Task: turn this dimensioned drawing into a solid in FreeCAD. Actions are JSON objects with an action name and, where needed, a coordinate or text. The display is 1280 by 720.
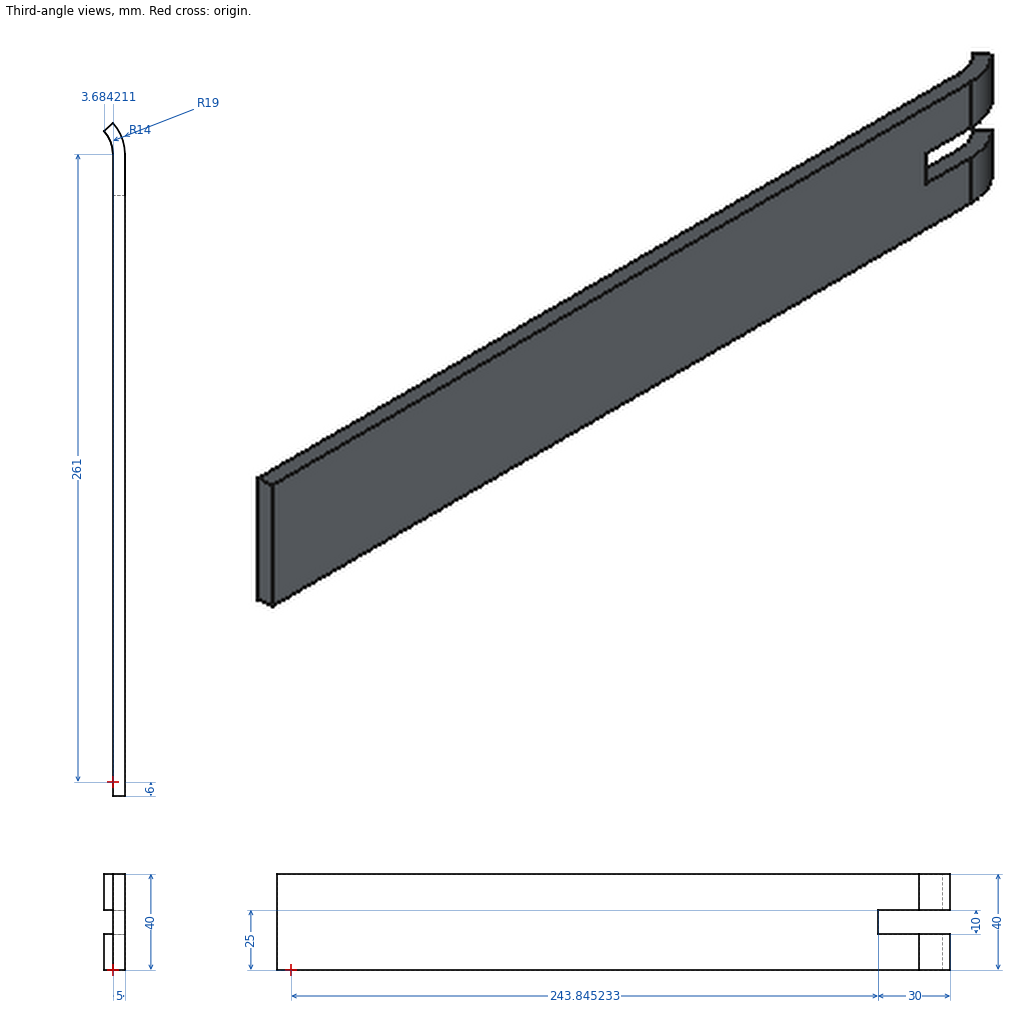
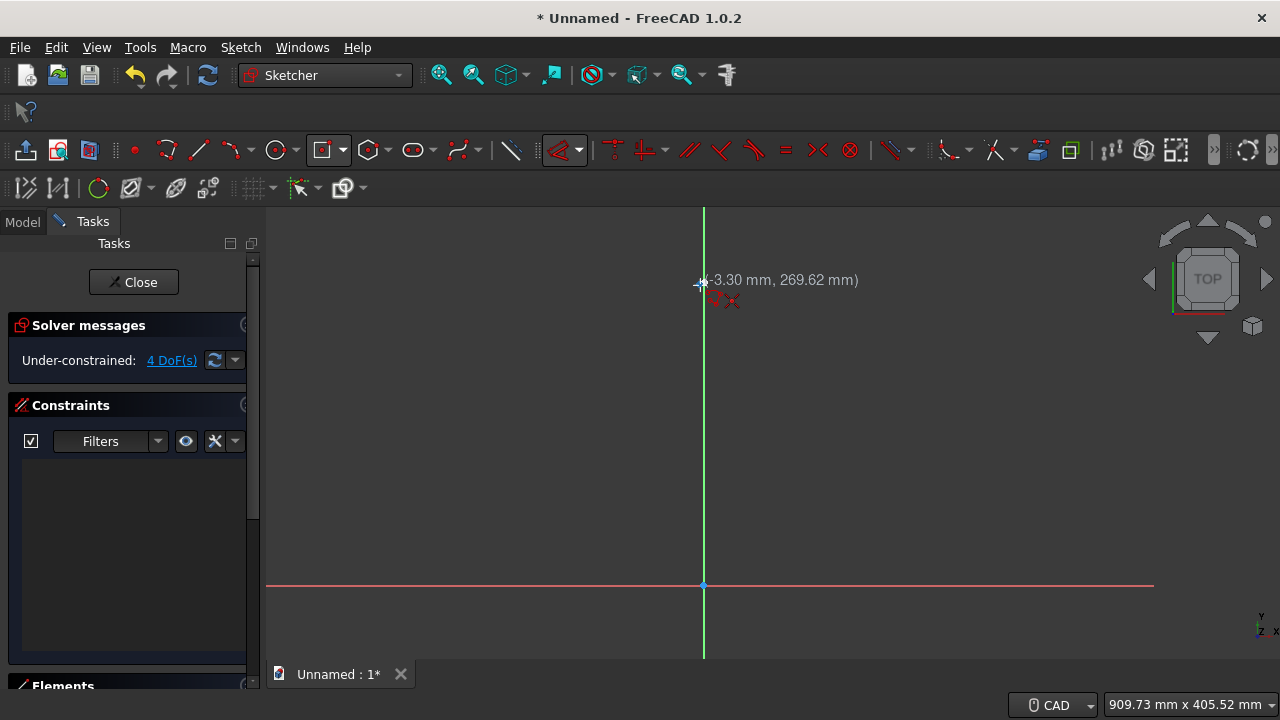
{"action": "scroll", "coordinate": [704, 295], "scroll_direction": "up", "scroll_amount": 2}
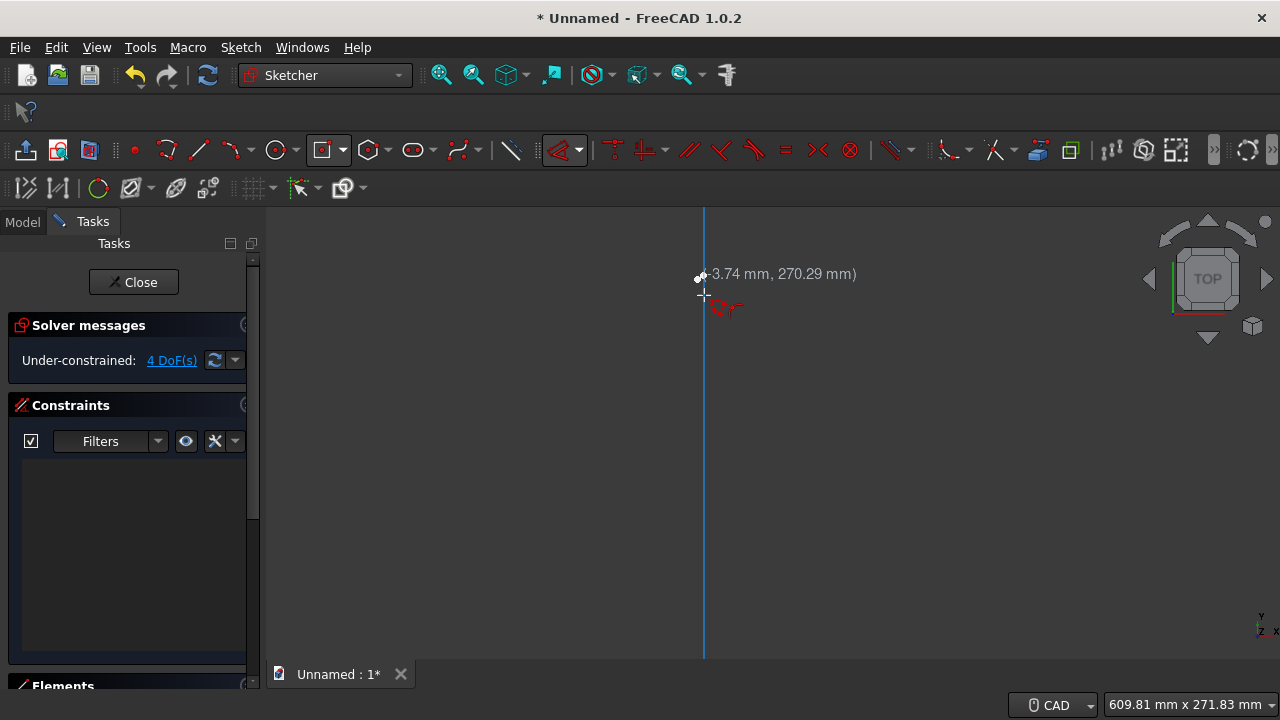
{"action": "left_click", "coordinate": [704, 295]}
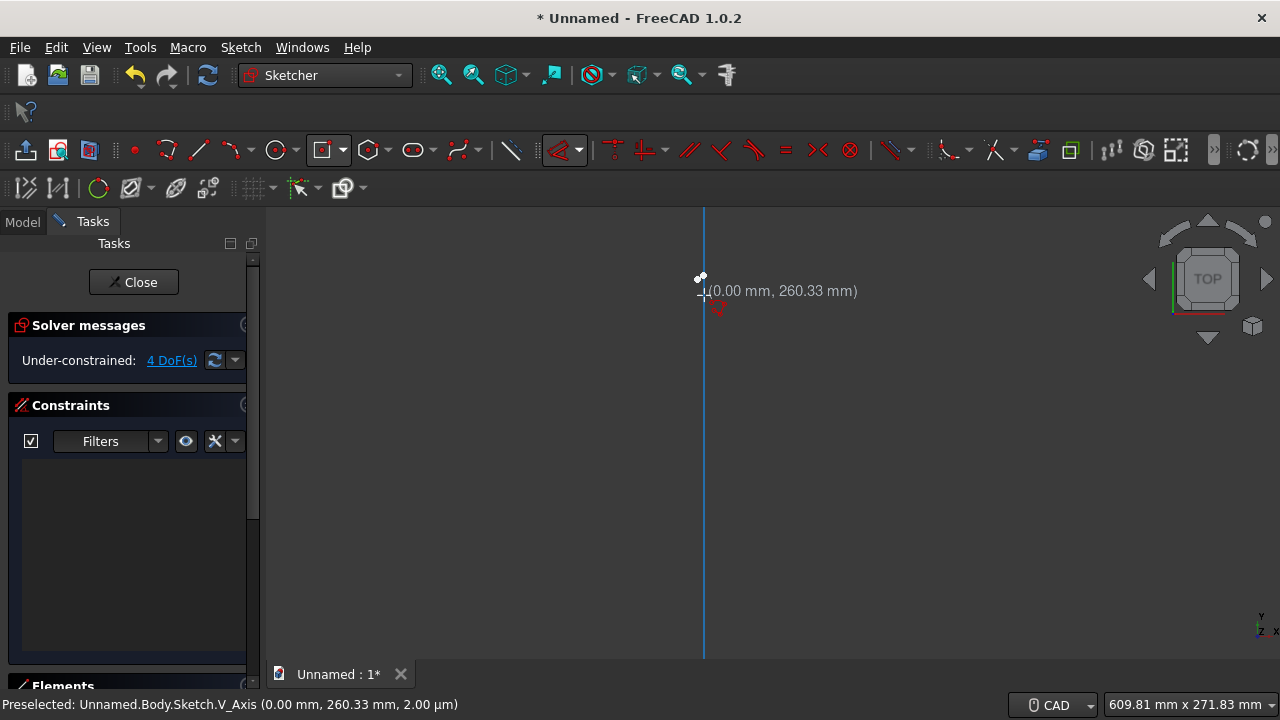
{"action": "scroll", "coordinate": [704, 294], "scroll_direction": "down", "scroll_amount": 2}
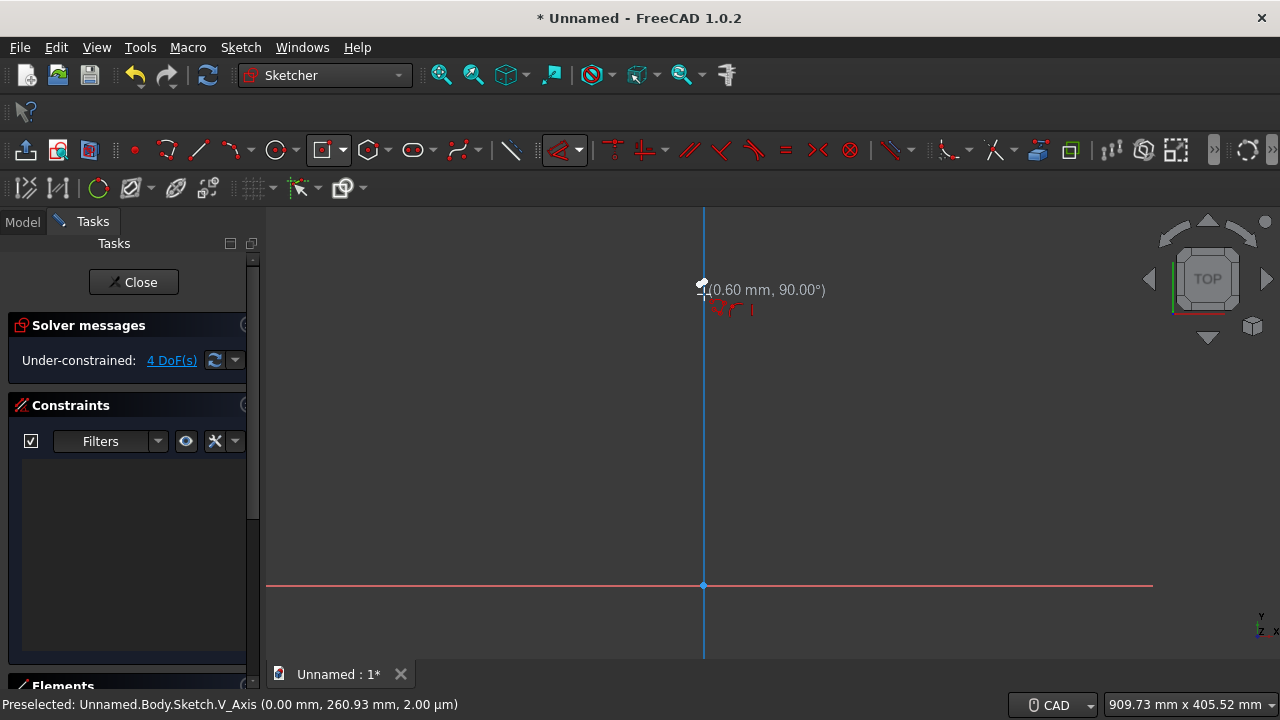
{"action": "left_click", "coordinate": [704, 586]}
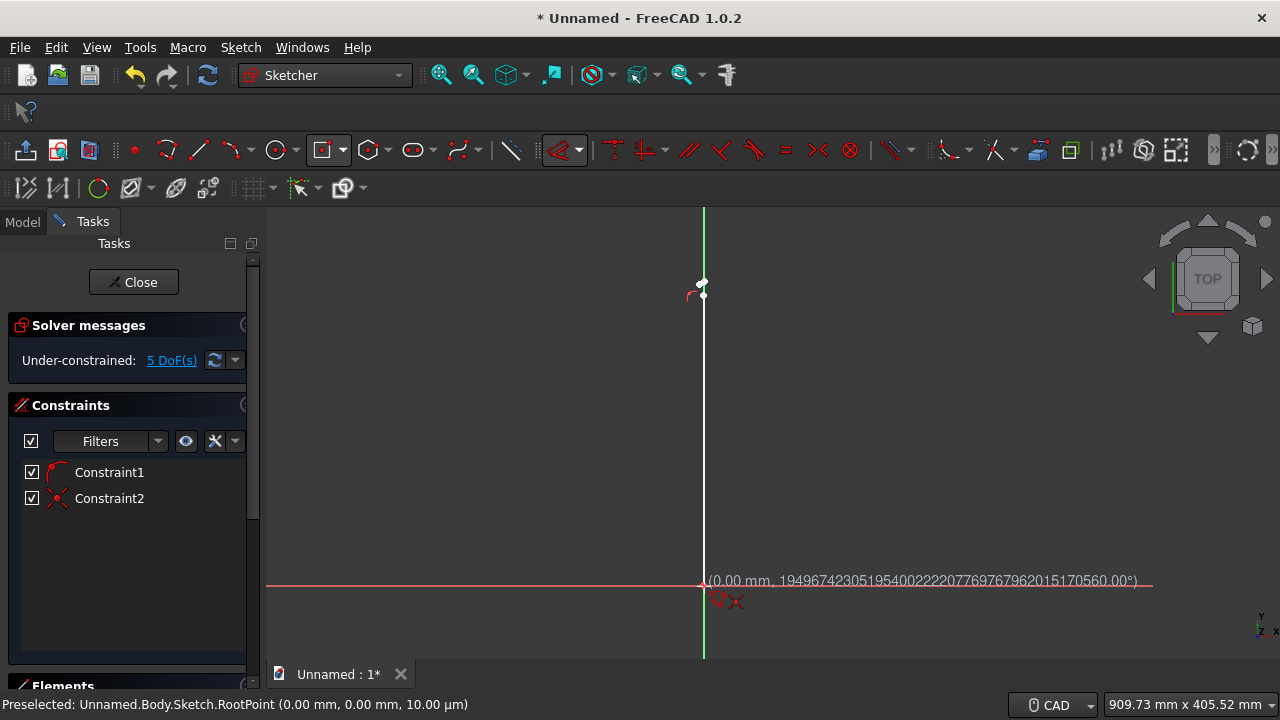
{"action": "scroll", "coordinate": [710, 586], "scroll_direction": "up", "scroll_amount": 6}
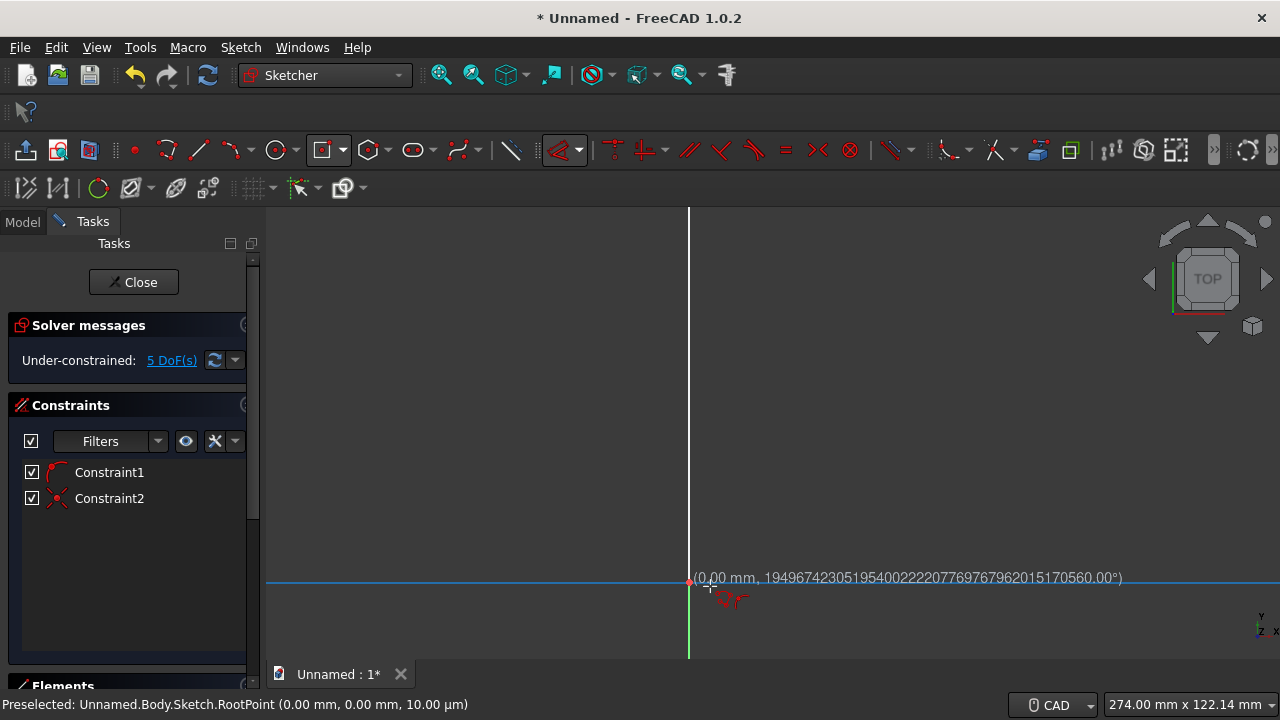
{"action": "left_click", "coordinate": [708, 574]}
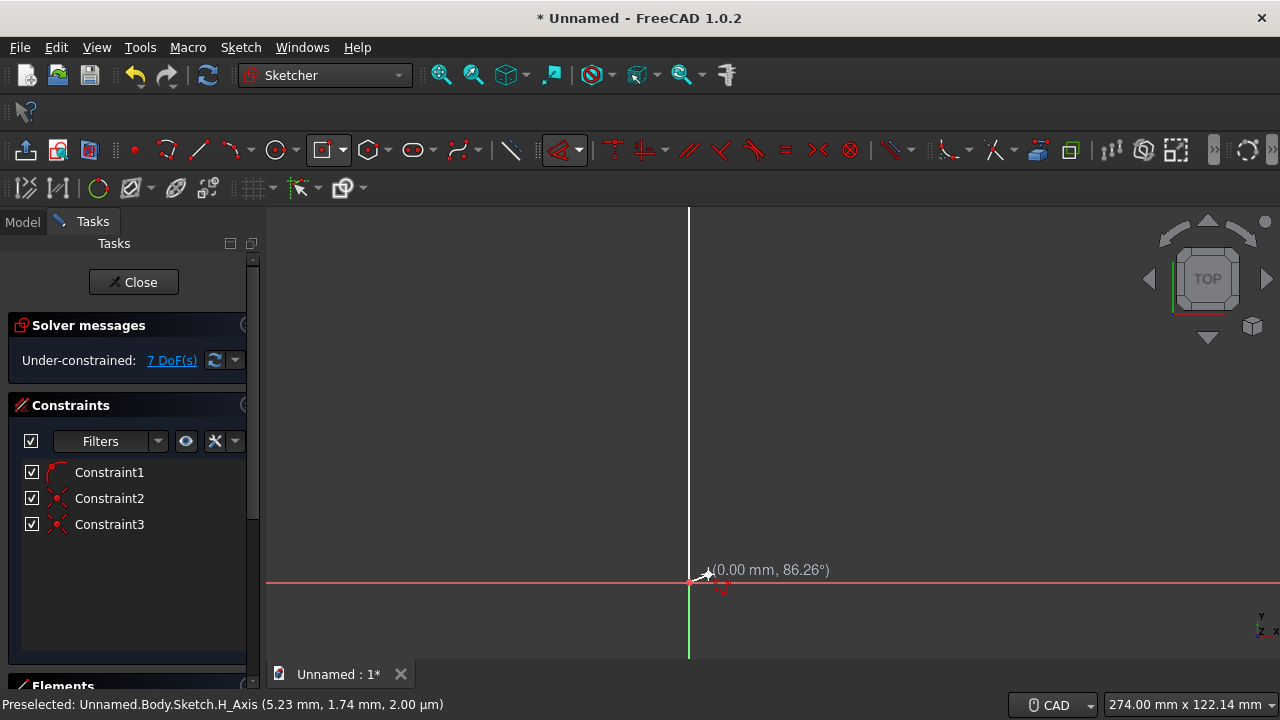
{"action": "scroll", "coordinate": [710, 587], "scroll_direction": "down", "scroll_amount": 6}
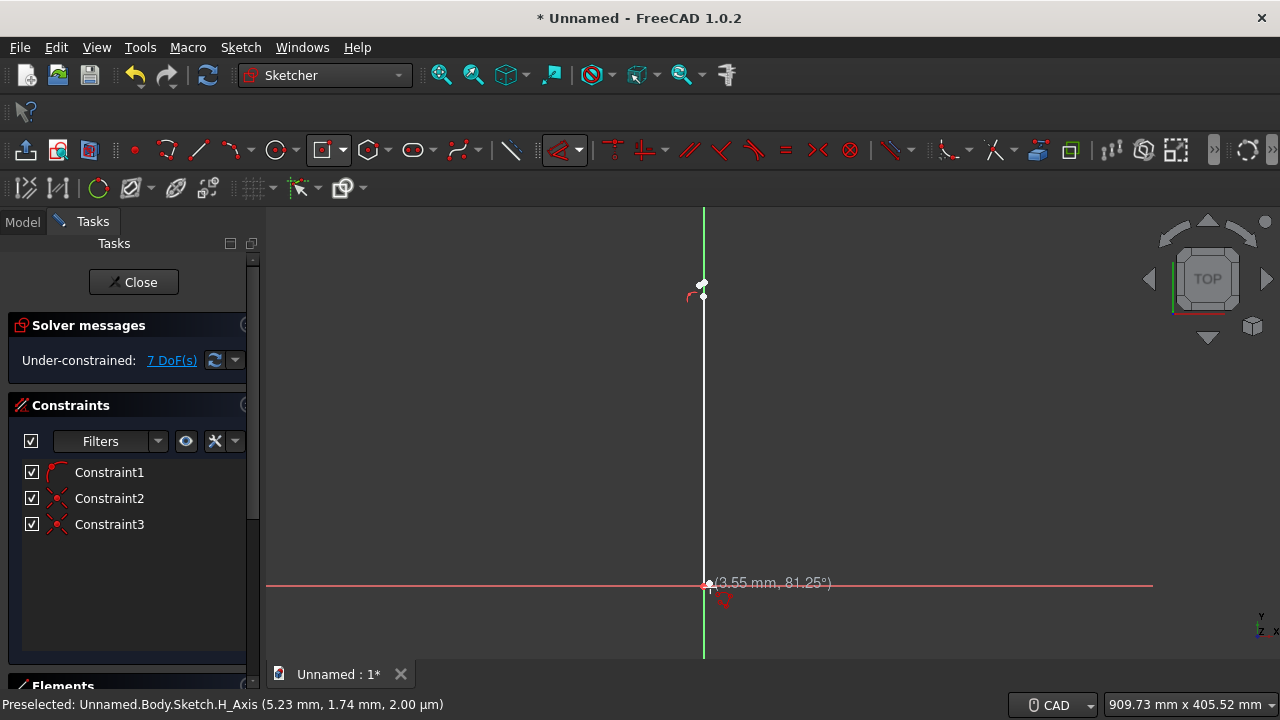
{"action": "scroll", "coordinate": [710, 295], "scroll_direction": "up", "scroll_amount": 6}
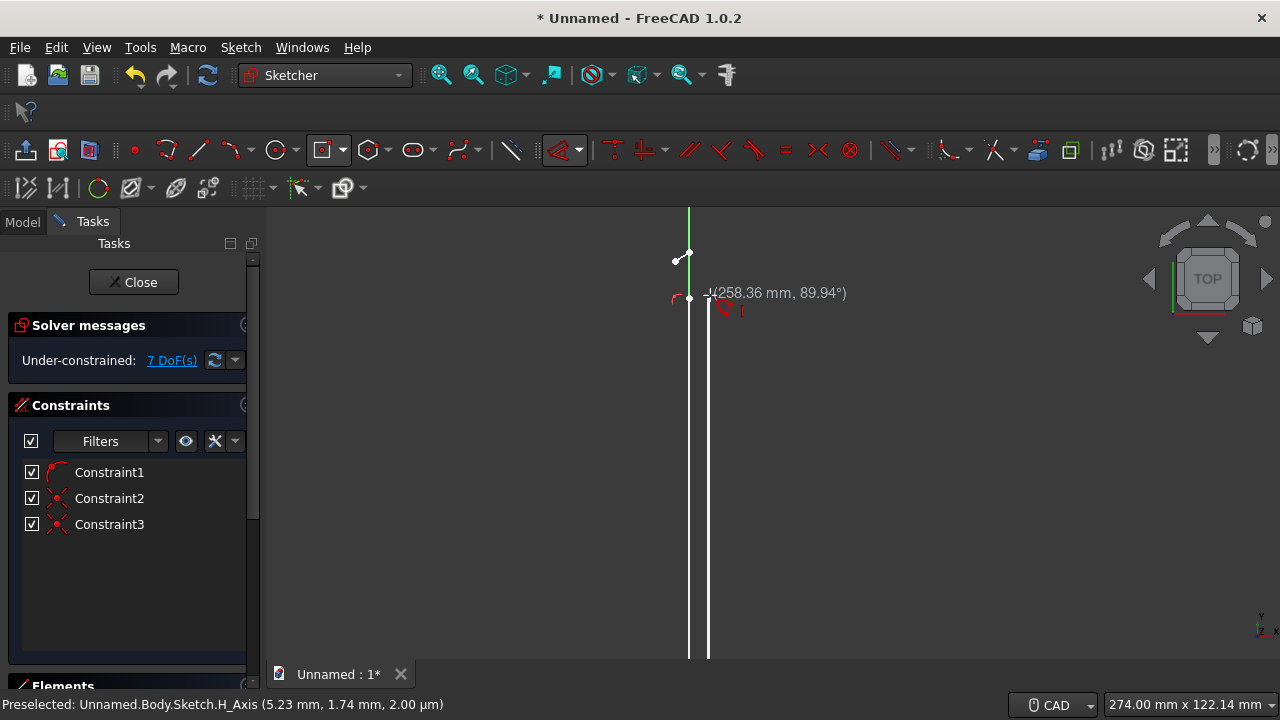
{"action": "left_click", "coordinate": [708, 296]}
{"action": "right_click", "coordinate": [708, 296]}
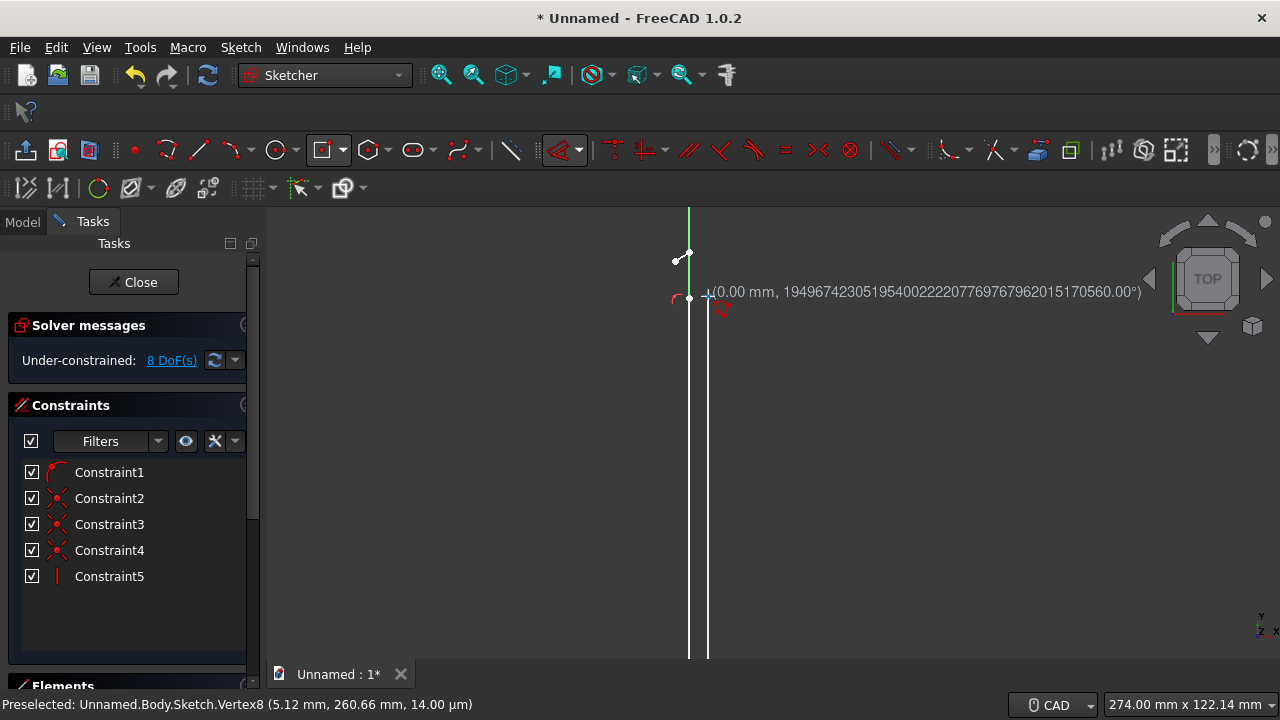
{"action": "left_click", "coordinate": [232, 150]}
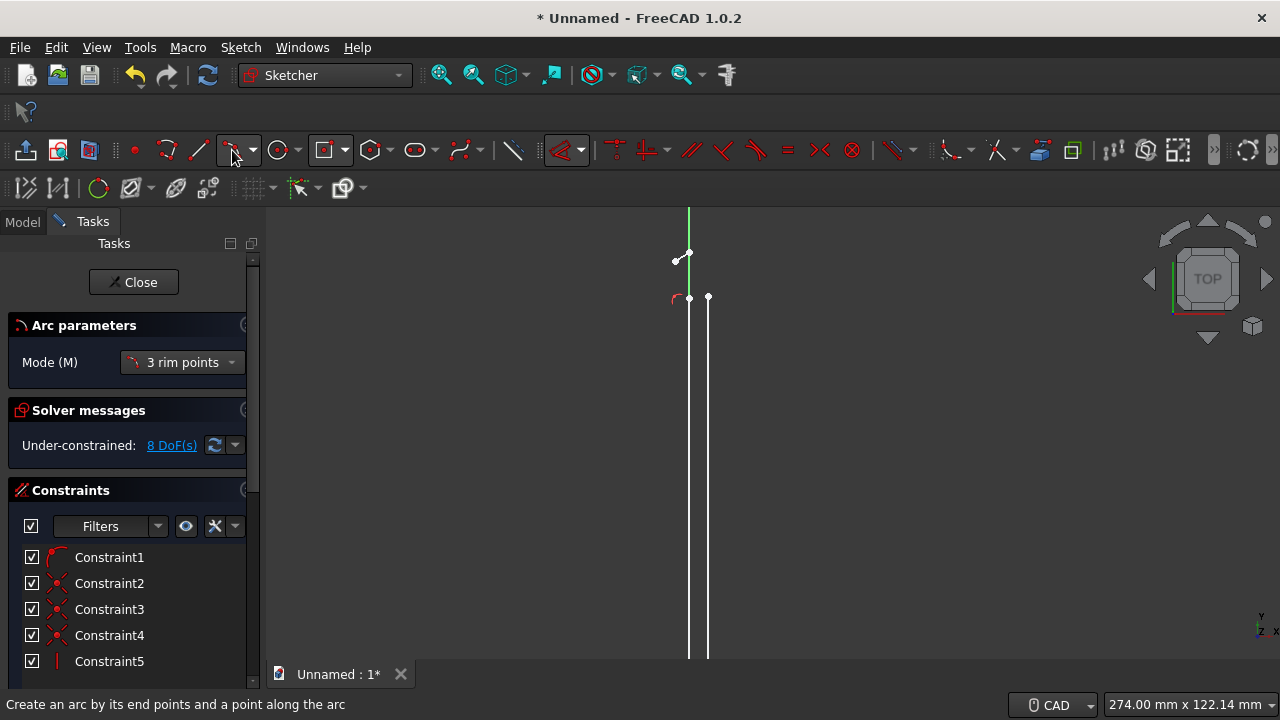
{"action": "scroll", "coordinate": [675, 261], "scroll_direction": "up", "scroll_amount": 3}